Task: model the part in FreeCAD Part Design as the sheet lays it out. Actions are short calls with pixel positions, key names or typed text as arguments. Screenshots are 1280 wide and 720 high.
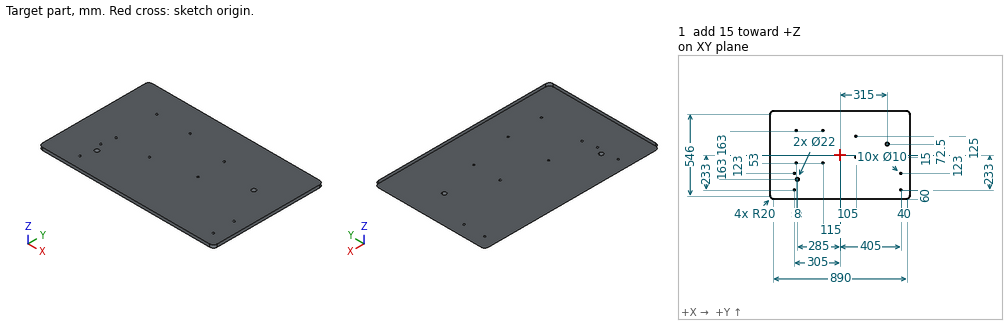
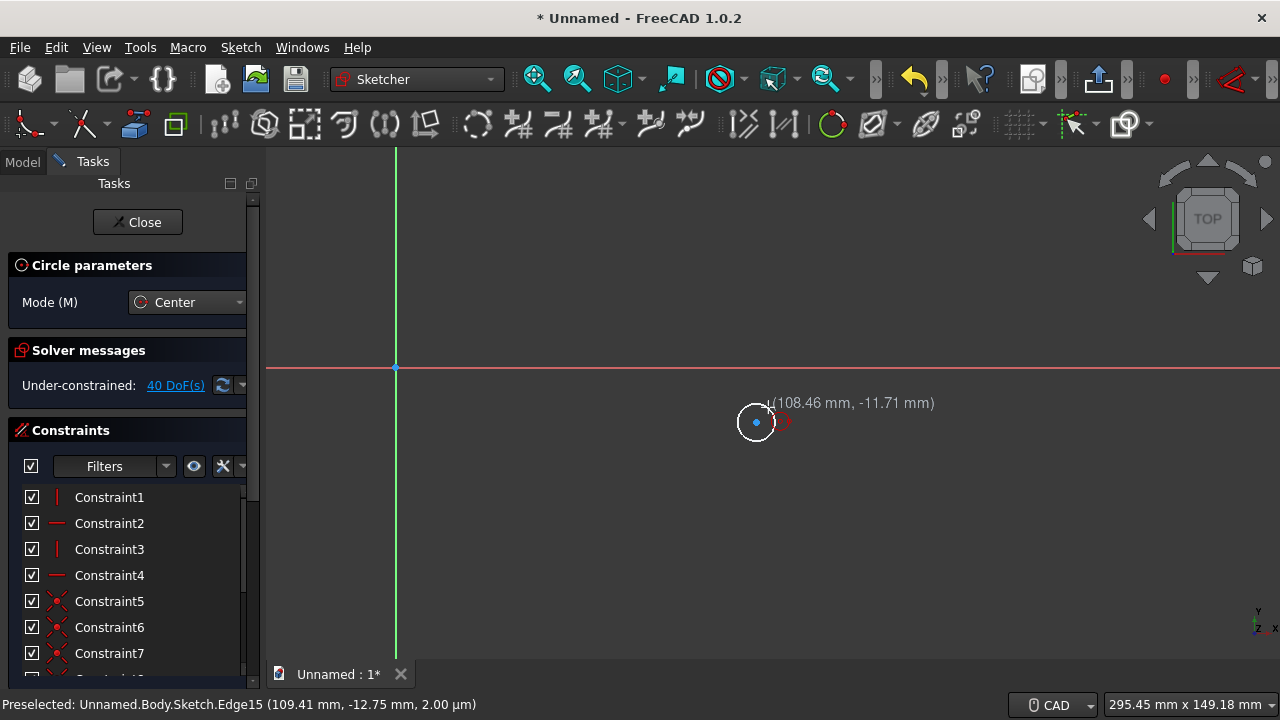
scroll(766, 410, down, 9)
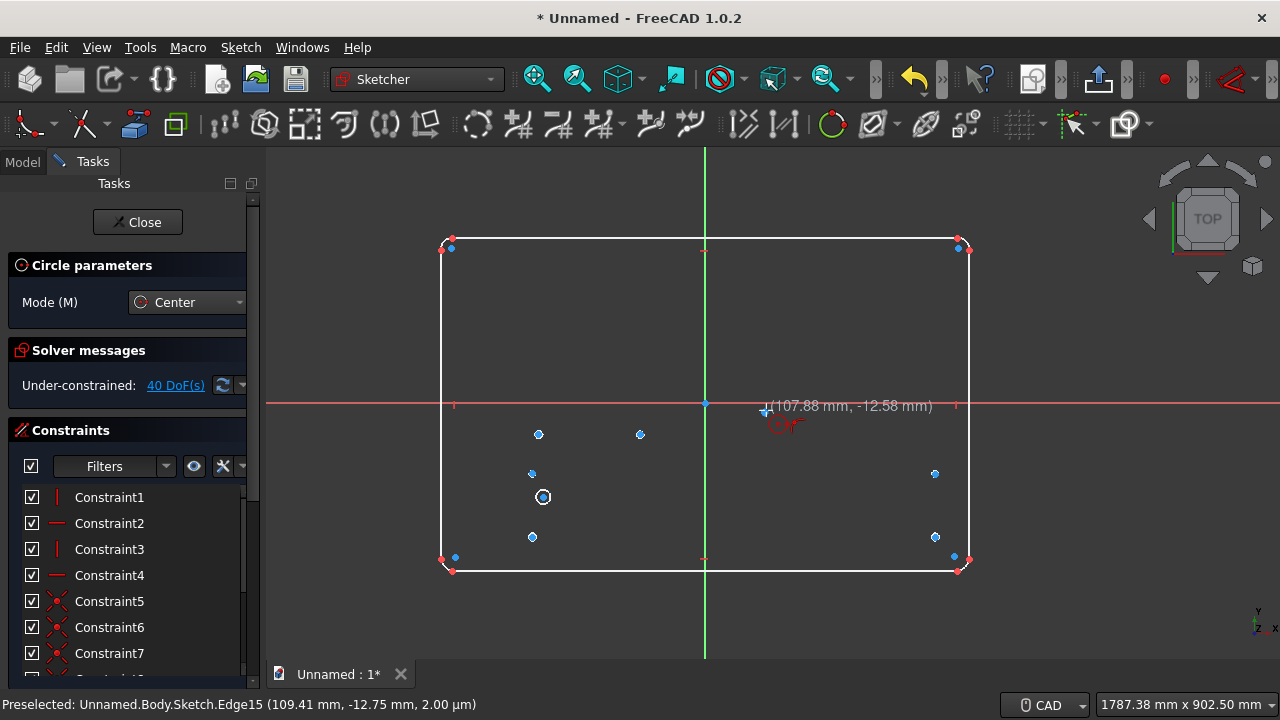
scroll(884, 362, up, 7)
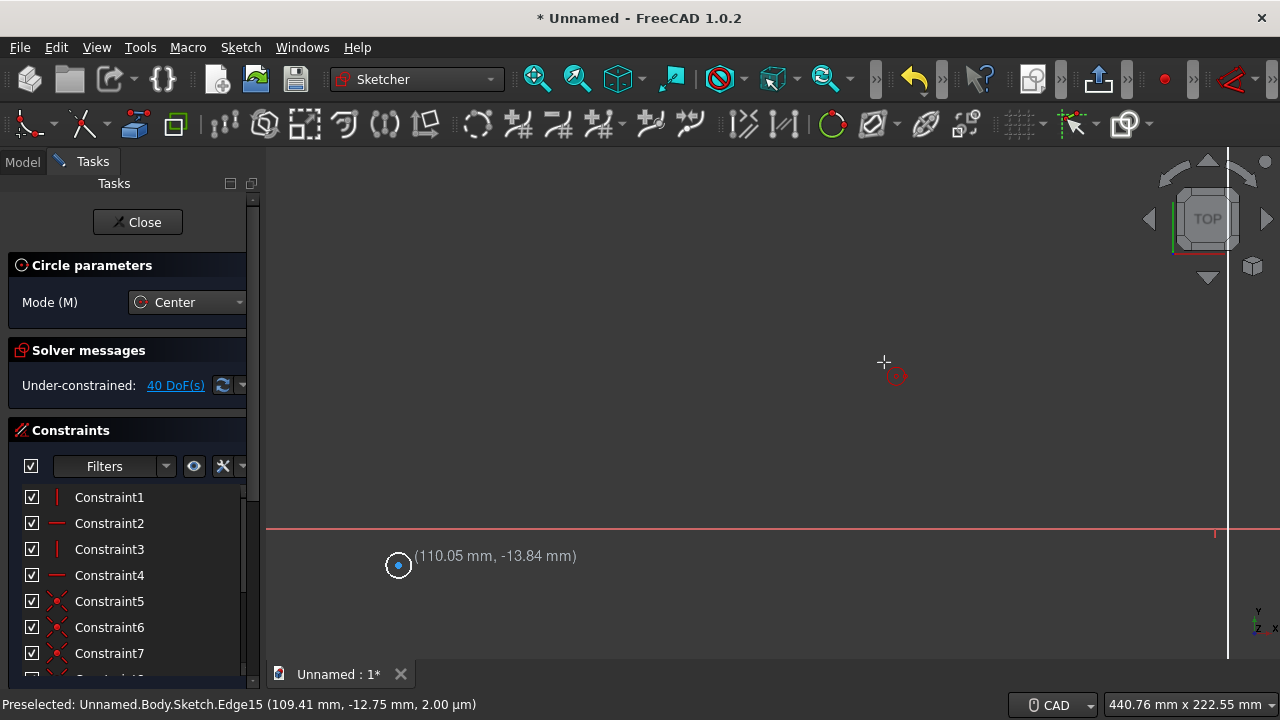
scroll(884, 362, down, 7)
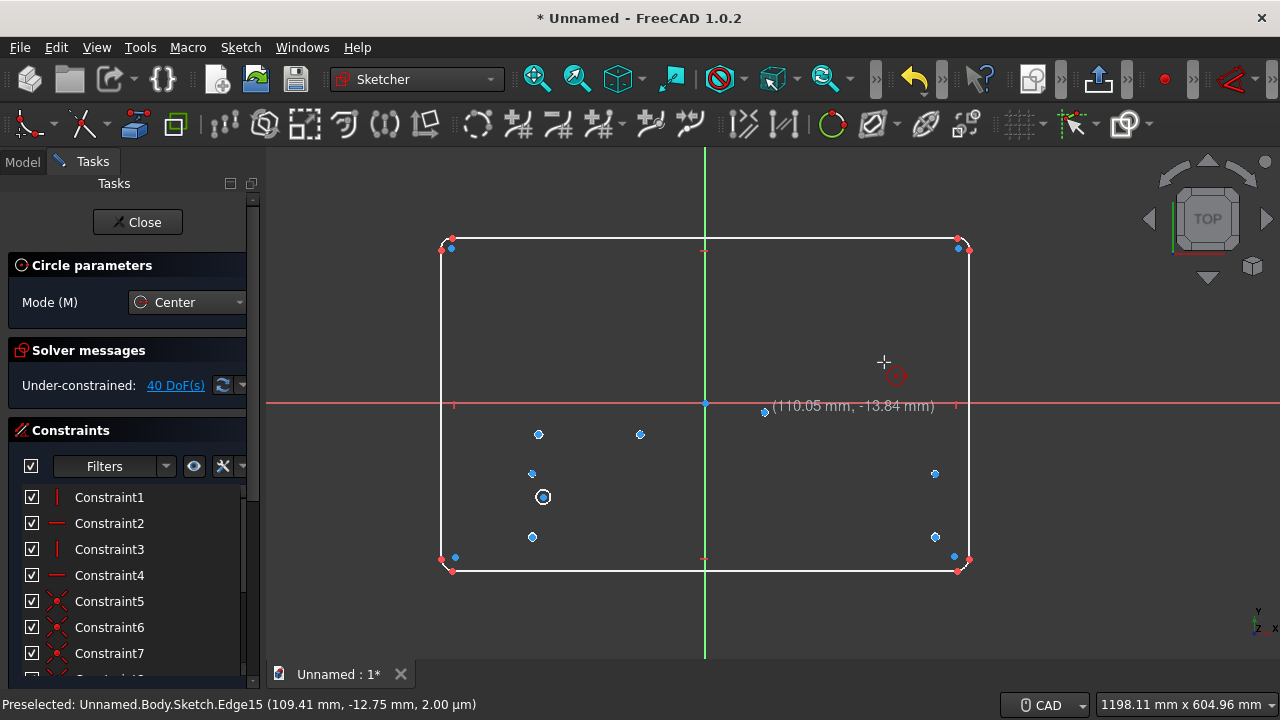
click(884, 362)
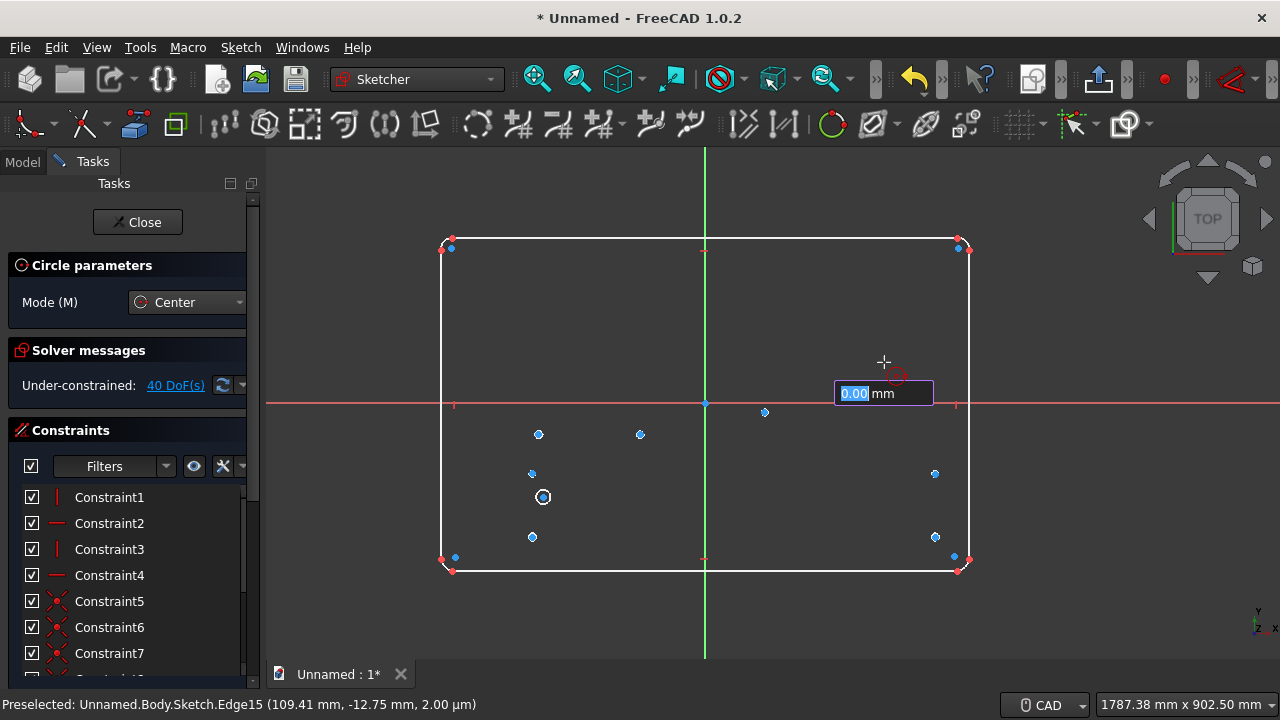
scroll(888, 358, up, 5)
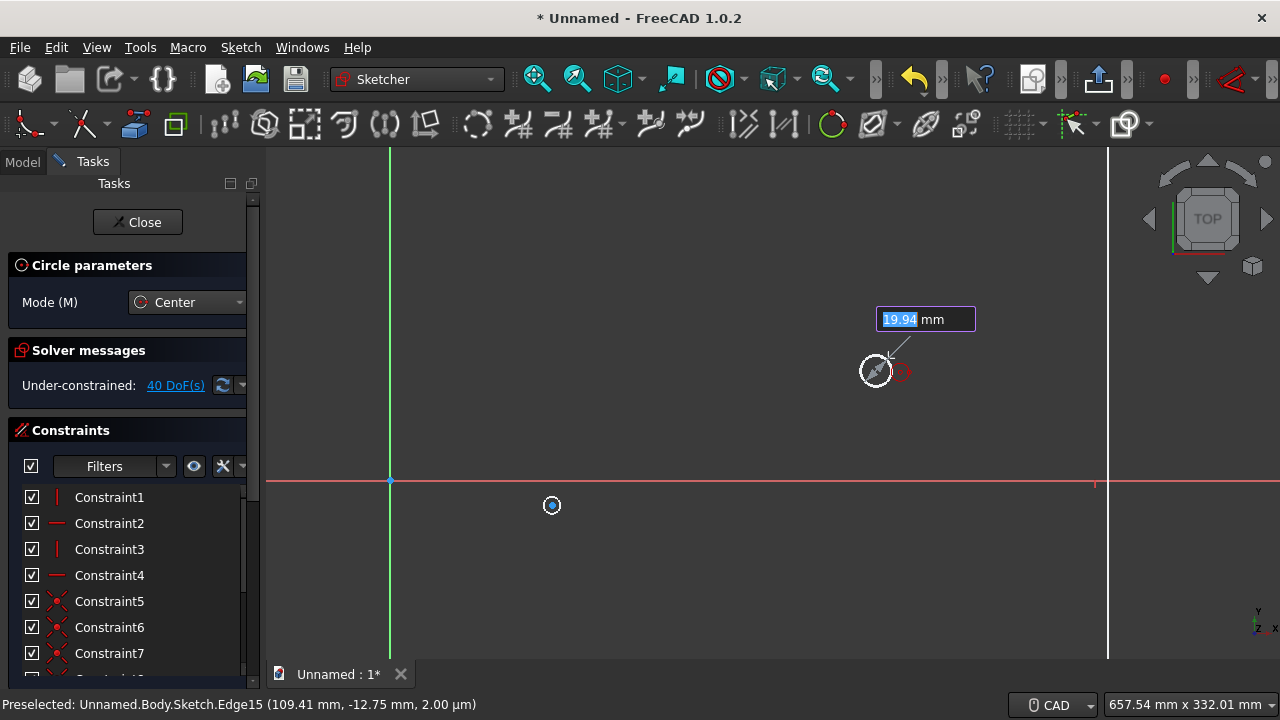
click(888, 357)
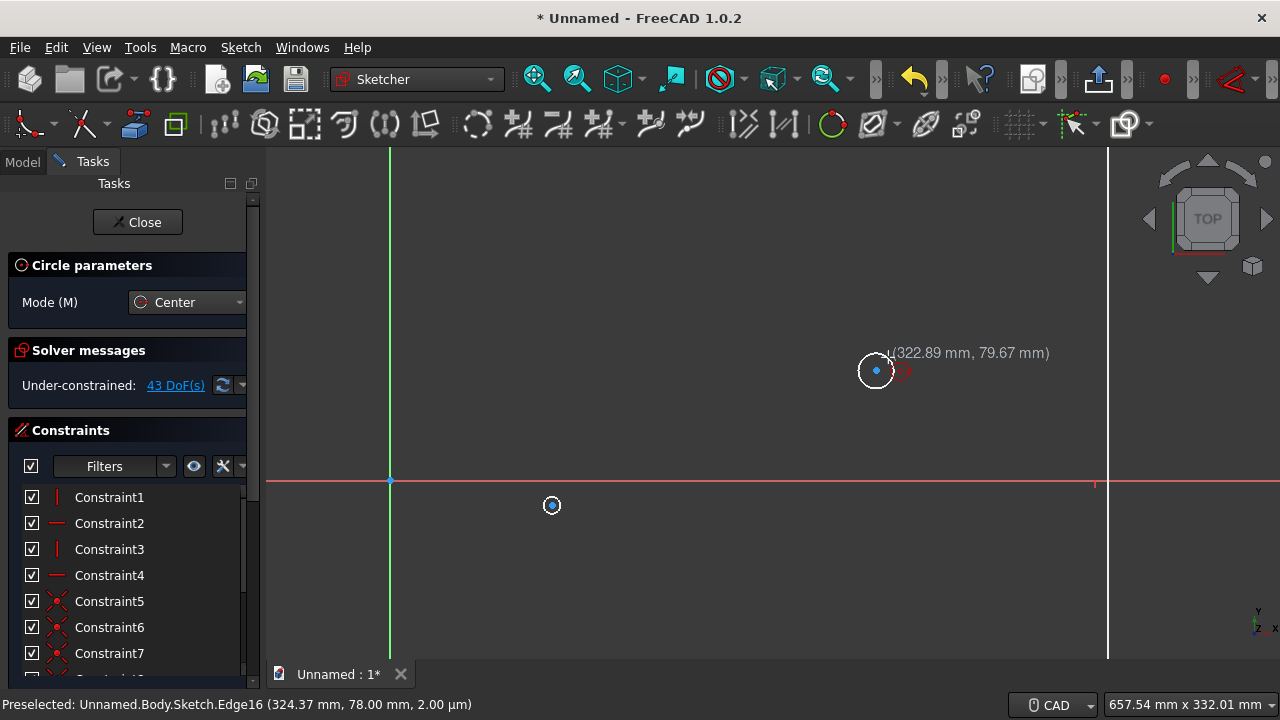
scroll(552, 288, up, 6)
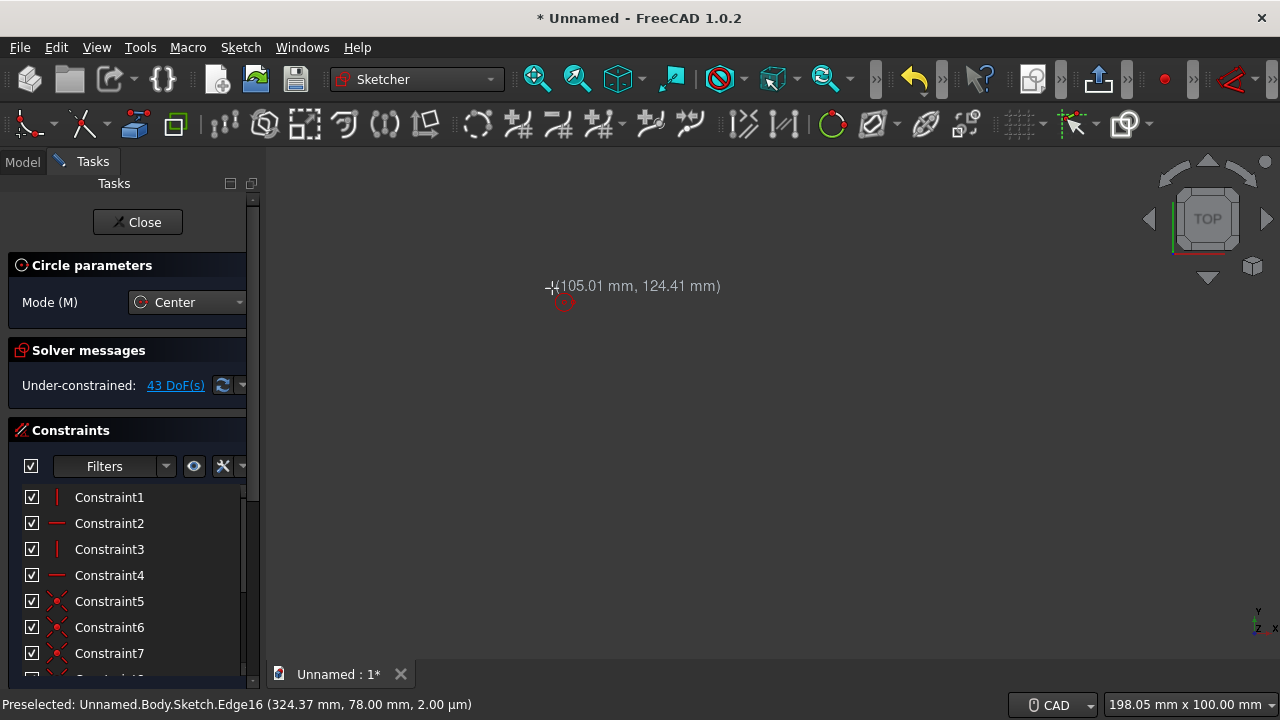
scroll(791, 338, down, 11)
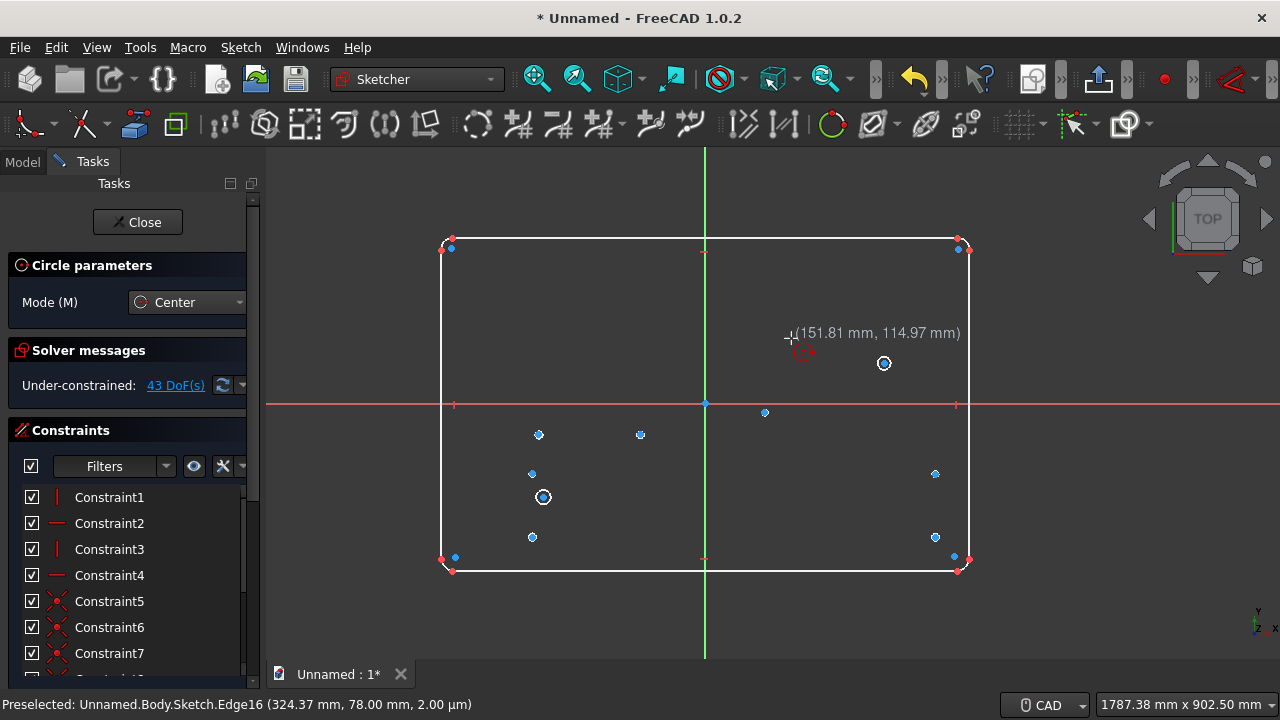
click(765, 333)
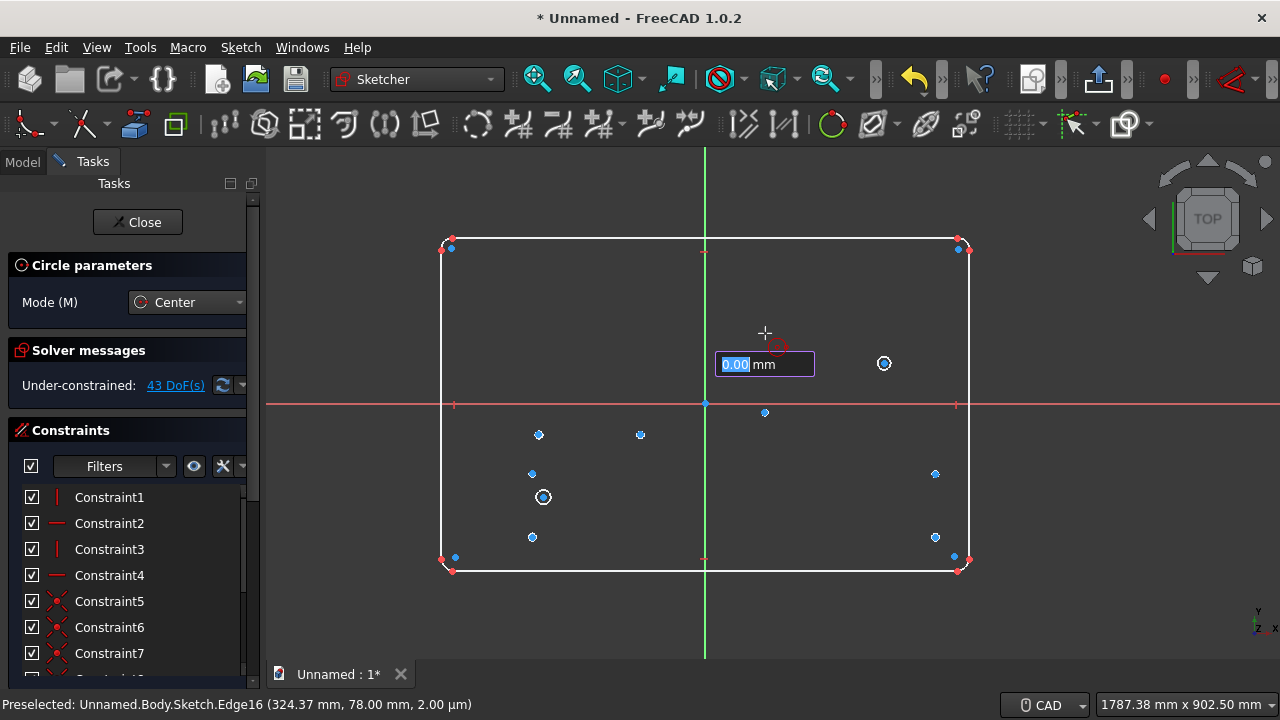
scroll(767, 331, up, 9)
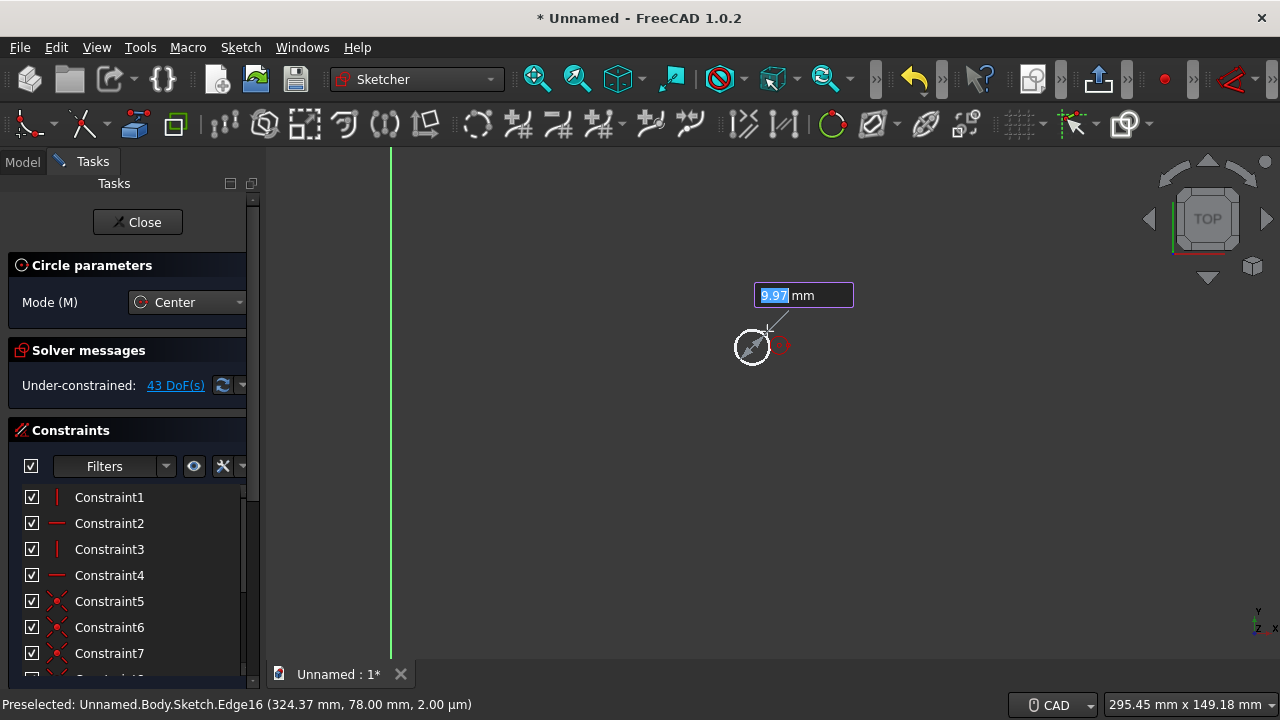
click(764, 328)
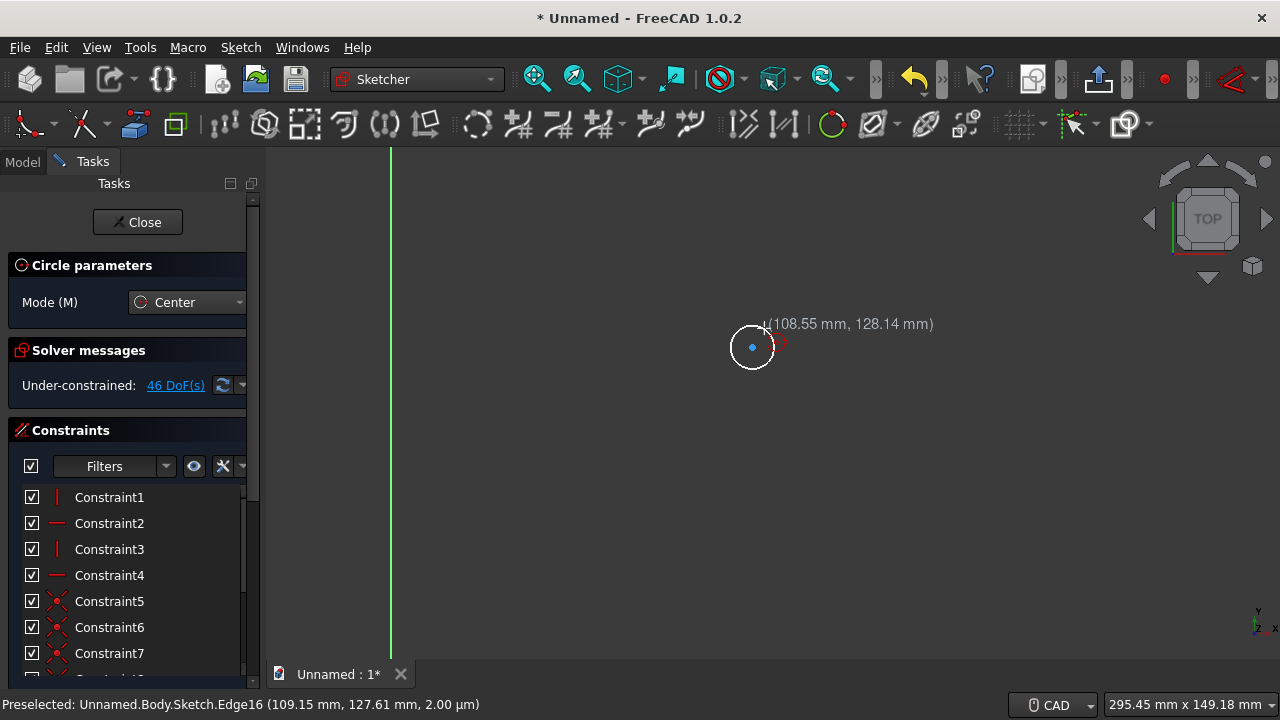
scroll(766, 331, down, 9)